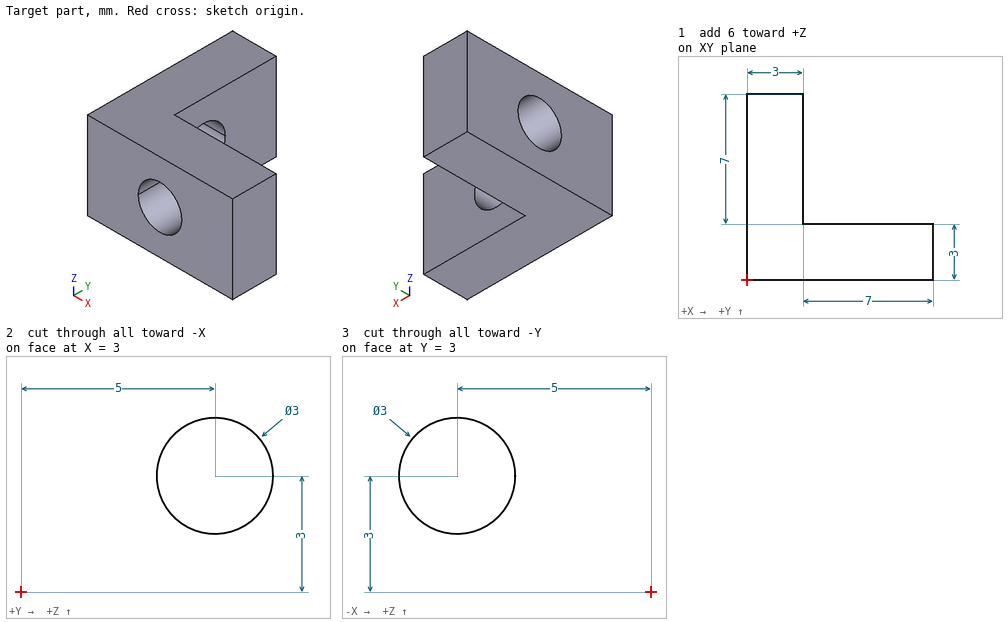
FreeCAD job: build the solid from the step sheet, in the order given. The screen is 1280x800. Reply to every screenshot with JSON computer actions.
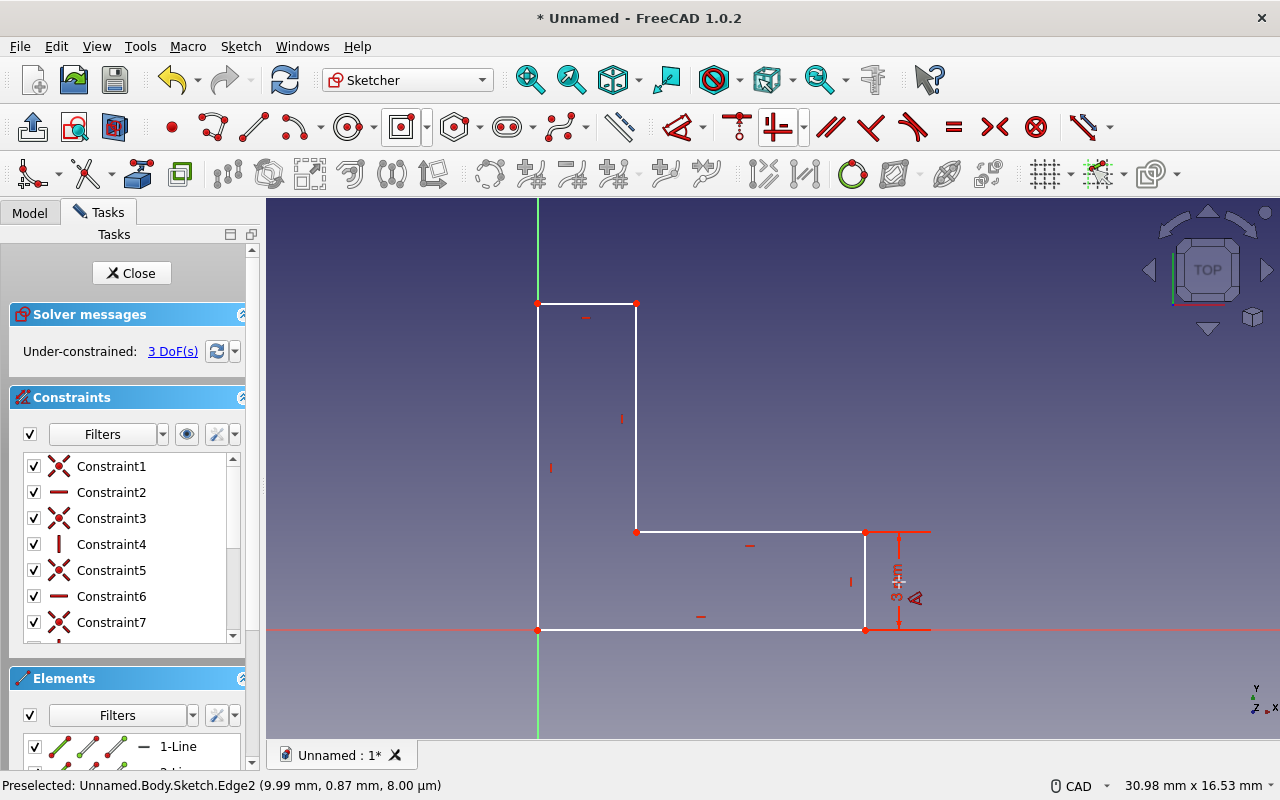
{"action": "left_click", "coordinate": [796, 532]}
{"action": "left_click", "coordinate": [751, 566]}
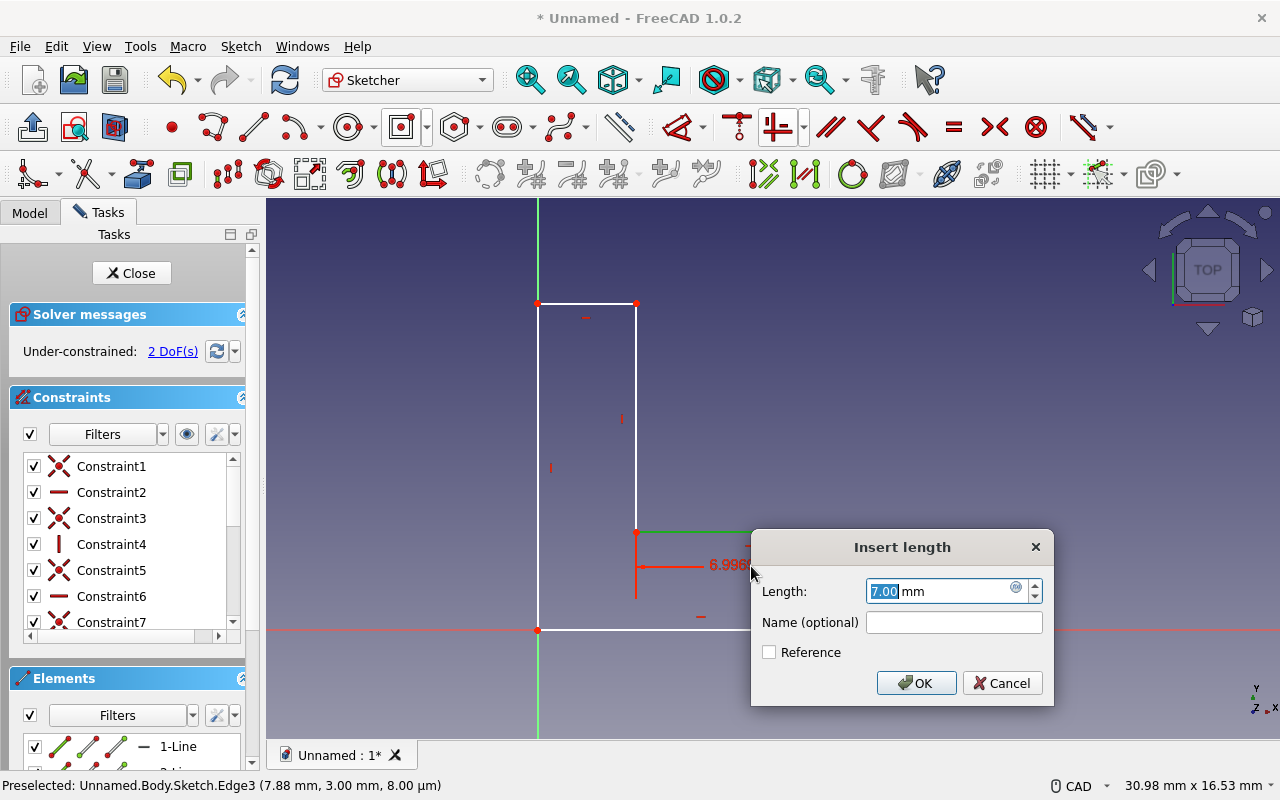
{"action": "type", "text": "7"}
{"action": "key", "text": "Return"}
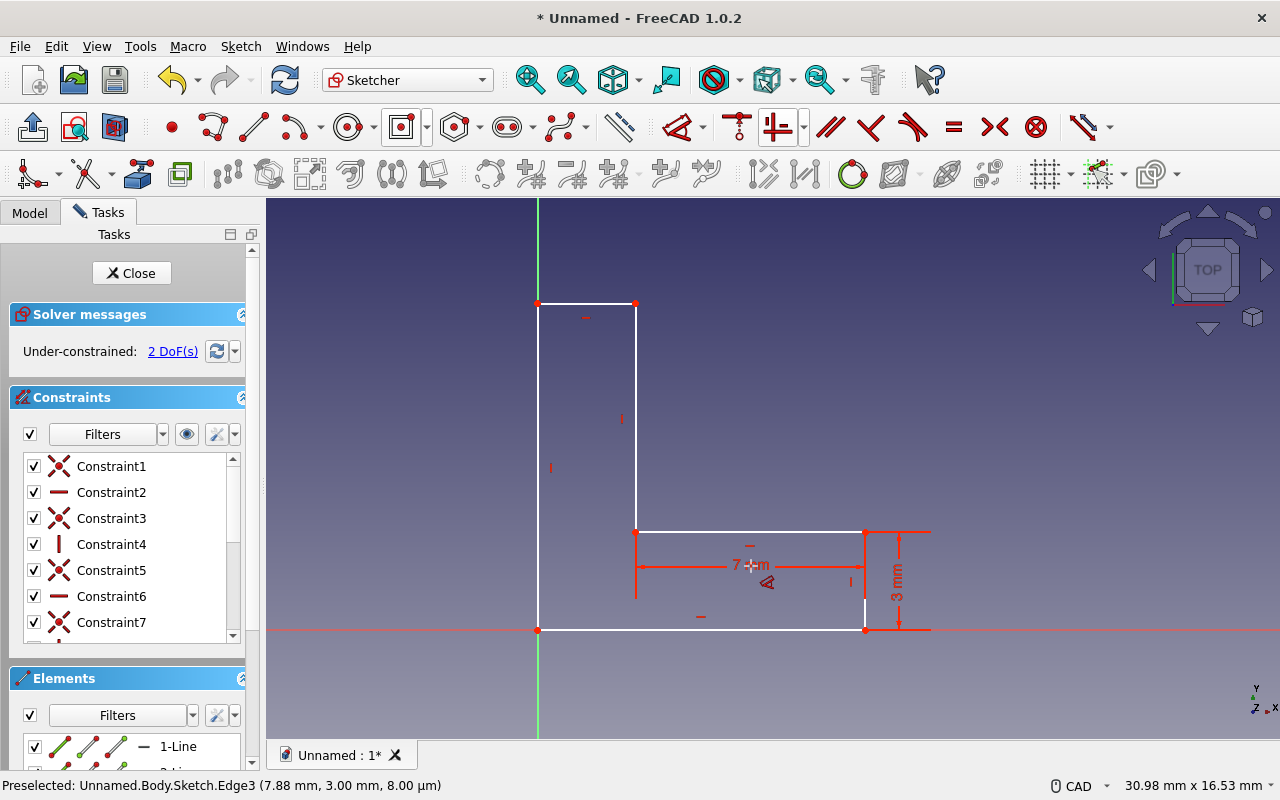
{"action": "left_click", "coordinate": [636, 464]}
{"action": "left_click", "coordinate": [602, 418]}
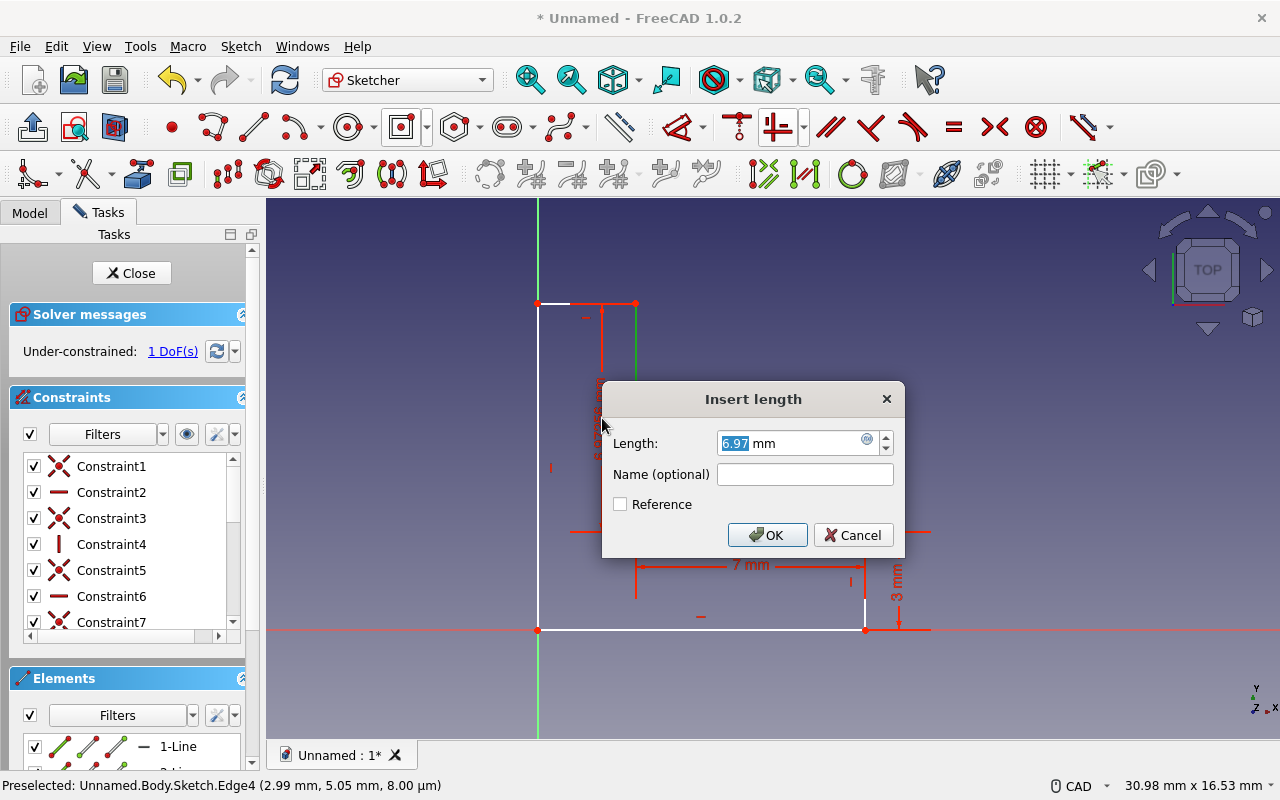
{"action": "type", "text": "7"}
{"action": "key", "text": "Return"}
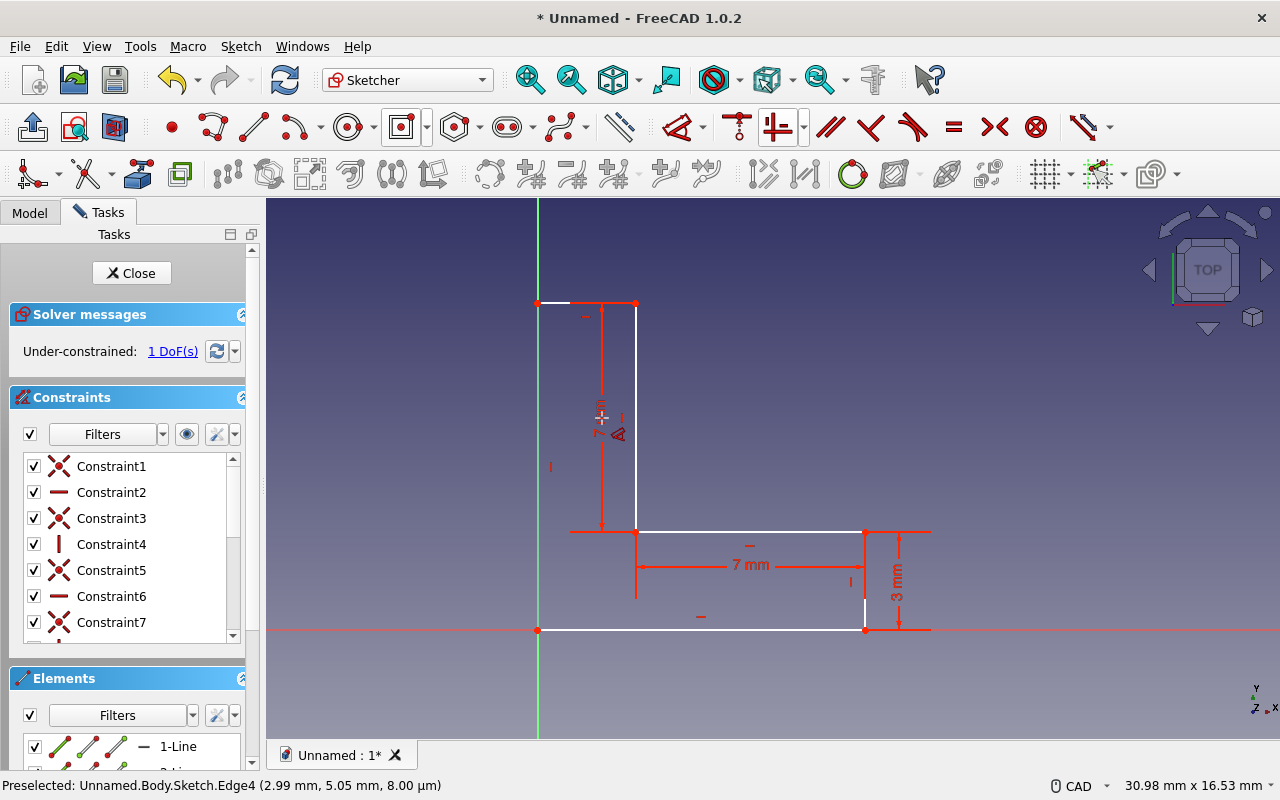
{"action": "left_click", "coordinate": [607, 303]}
{"action": "left_click", "coordinate": [587, 269]}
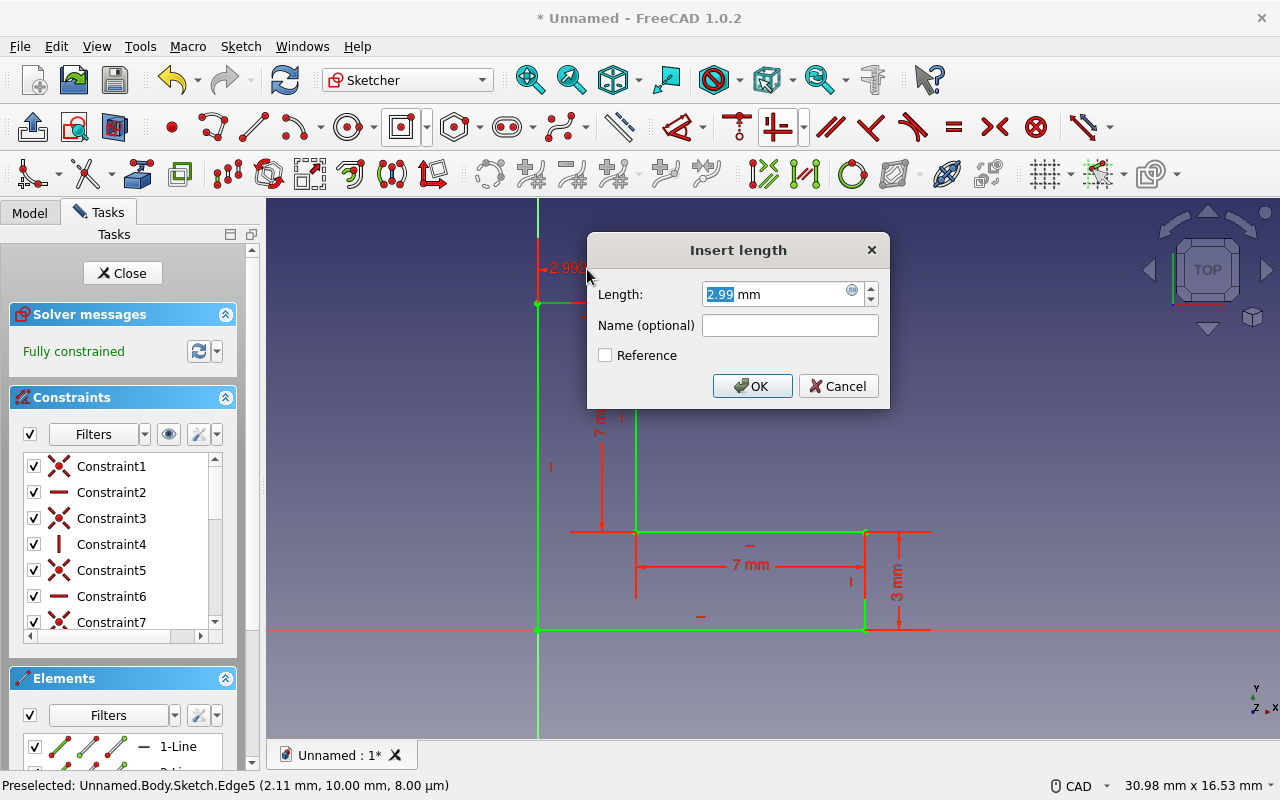
{"action": "type", "text": "3"}
{"action": "key", "text": "Return"}
{"action": "key", "text": "Escape"}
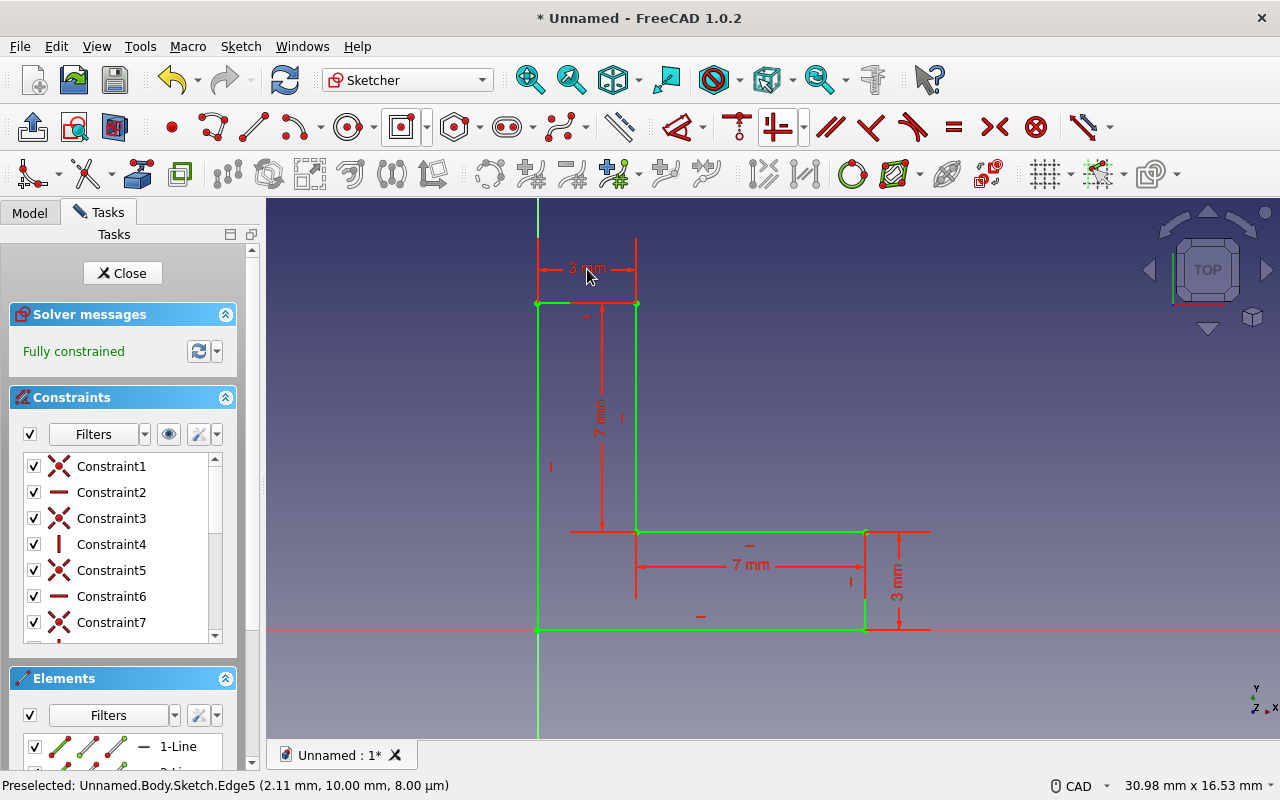
{"action": "left_click", "coordinate": [123, 273]}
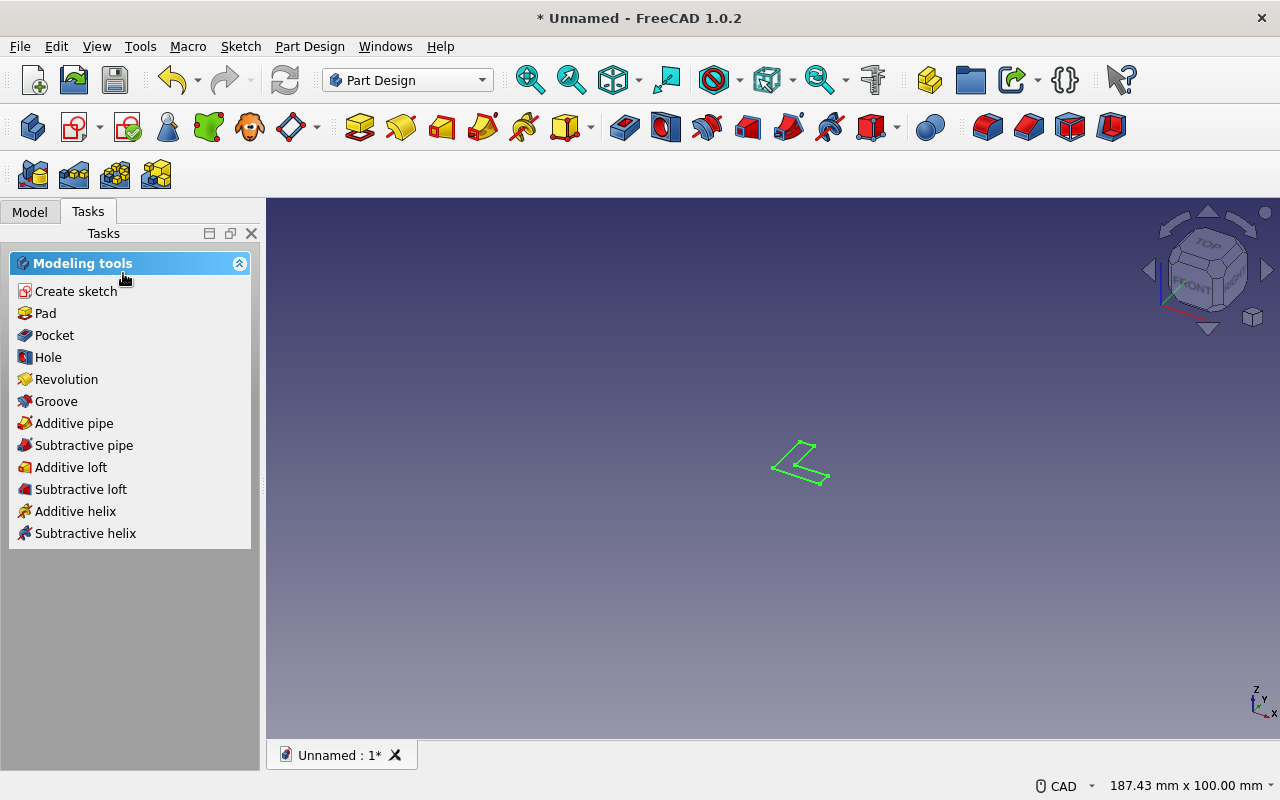
{"action": "left_click", "coordinate": [360, 128]}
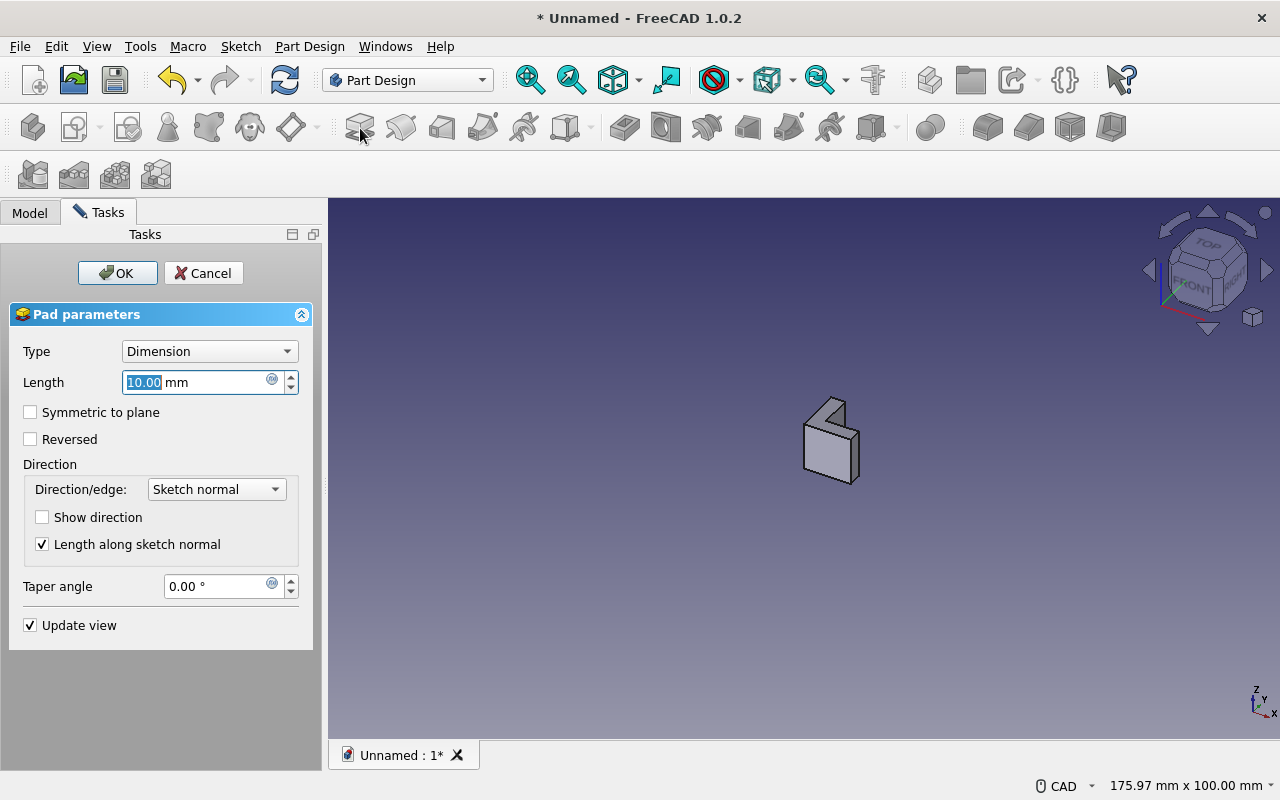
{"action": "type", "text": "6"}
{"action": "key", "text": "Tab"}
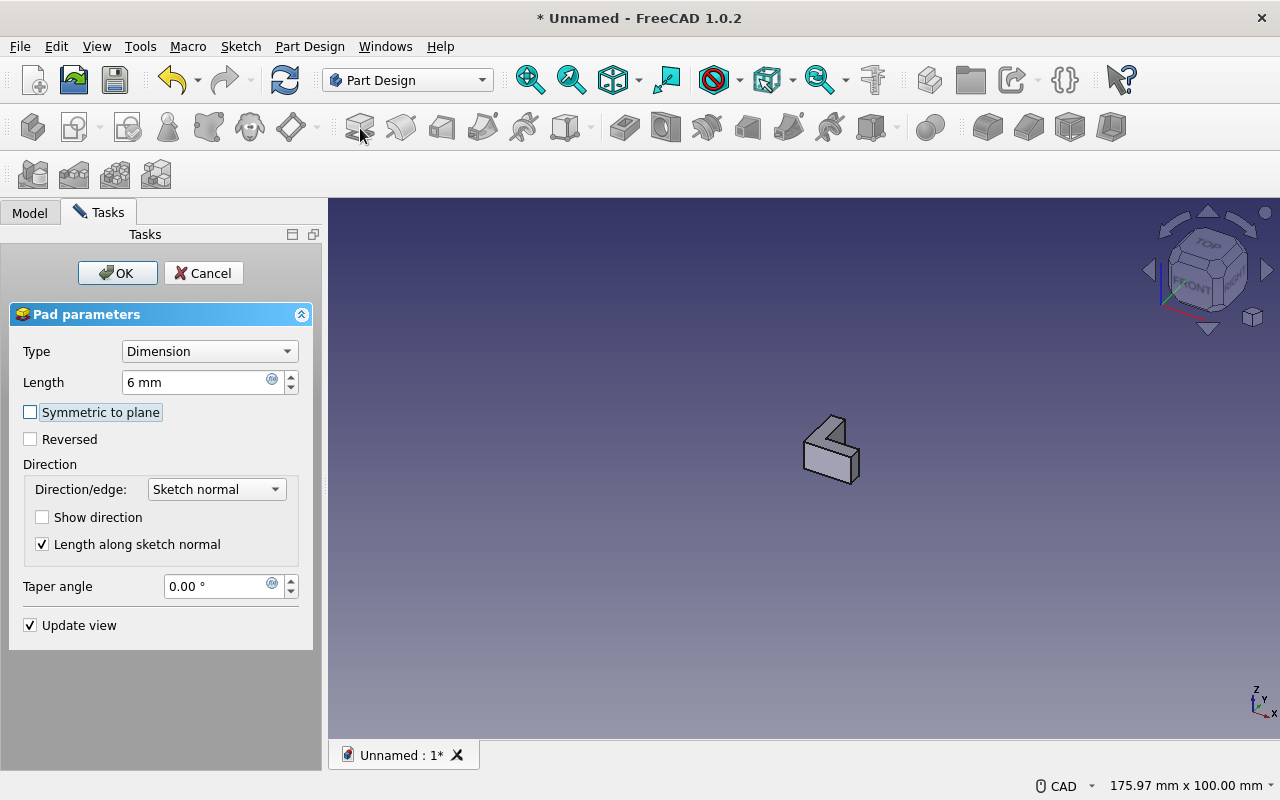
{"action": "left_click", "coordinate": [118, 273]}